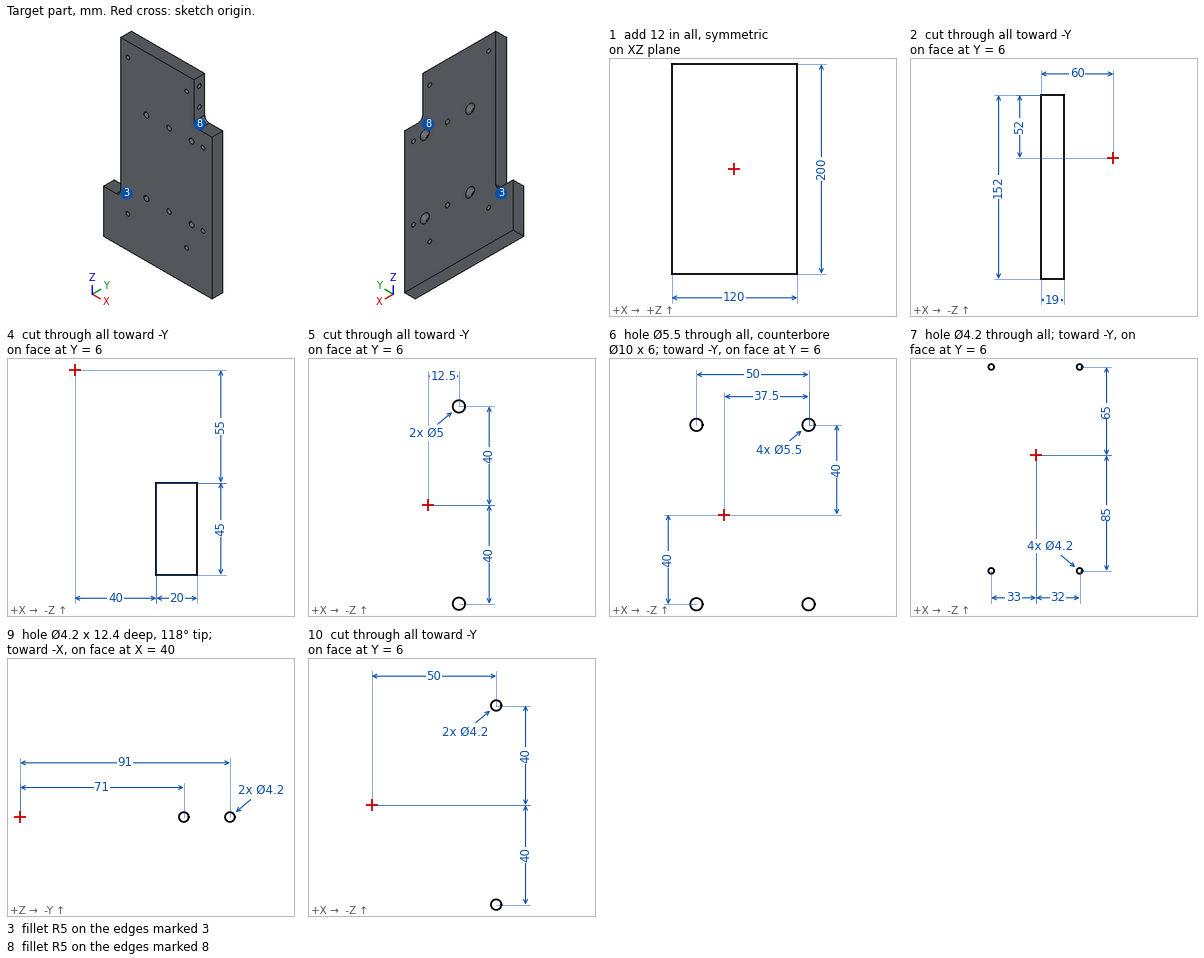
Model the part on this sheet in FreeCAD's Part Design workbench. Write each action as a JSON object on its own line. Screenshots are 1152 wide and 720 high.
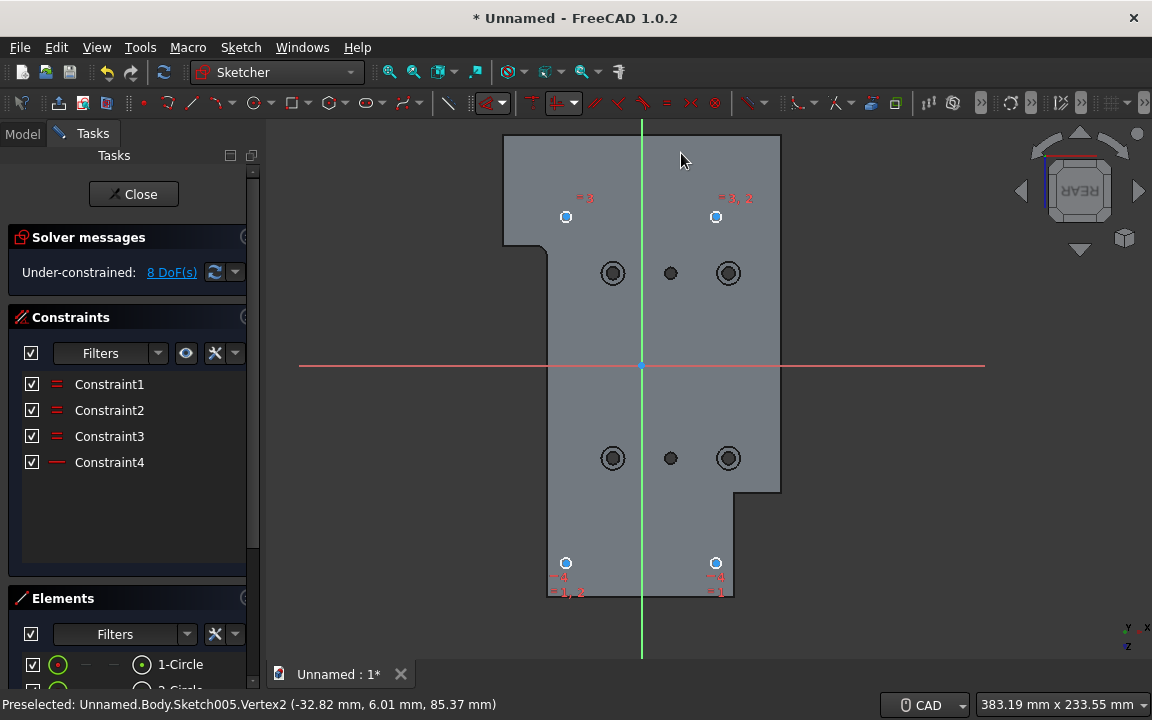
{"action": "left_click", "coordinate": [716, 563]}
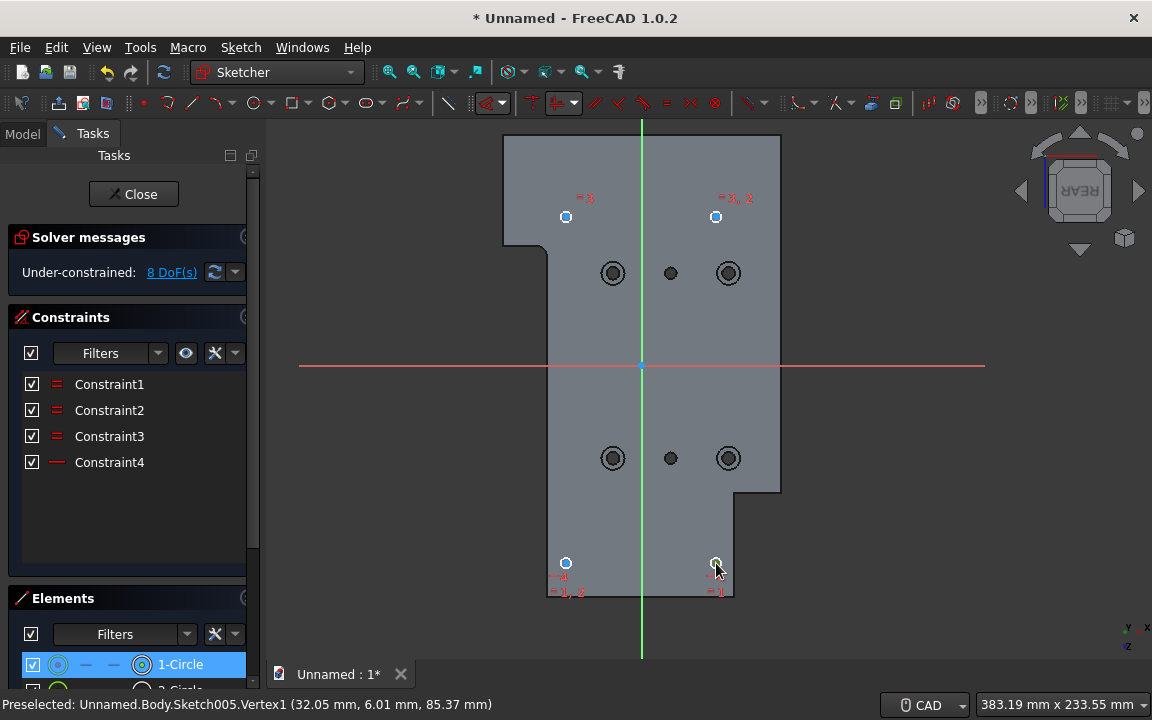
{"action": "left_click", "coordinate": [716, 217]}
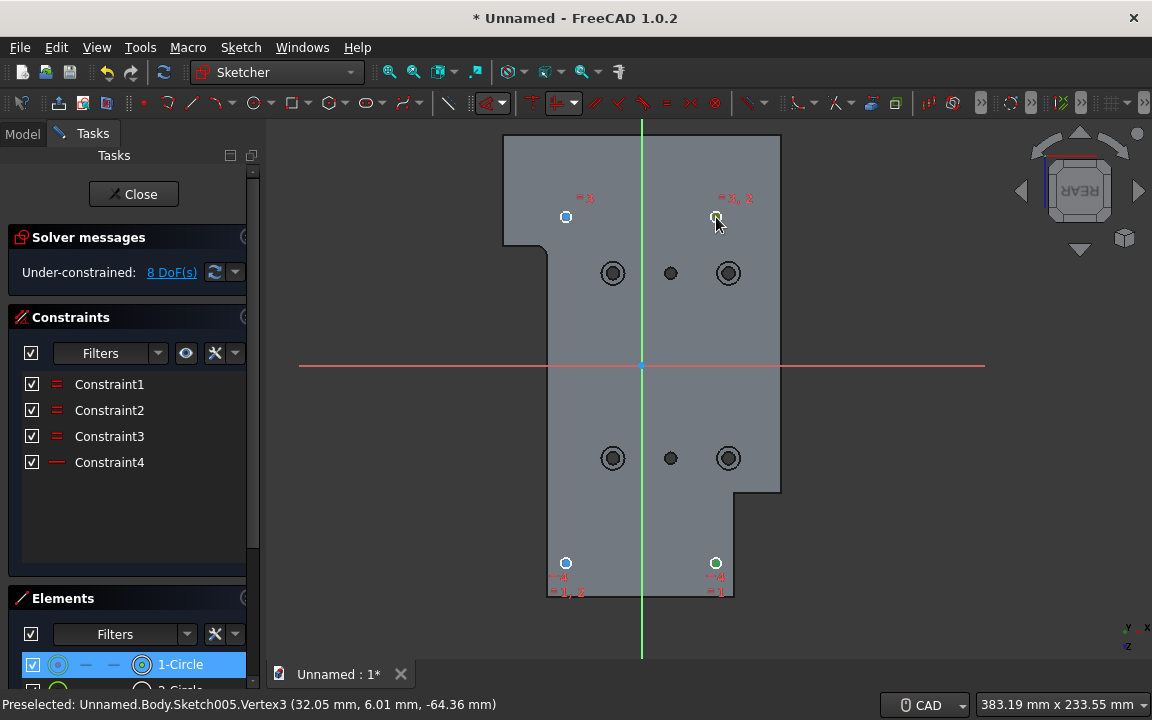
{"action": "left_click", "coordinate": [576, 104]}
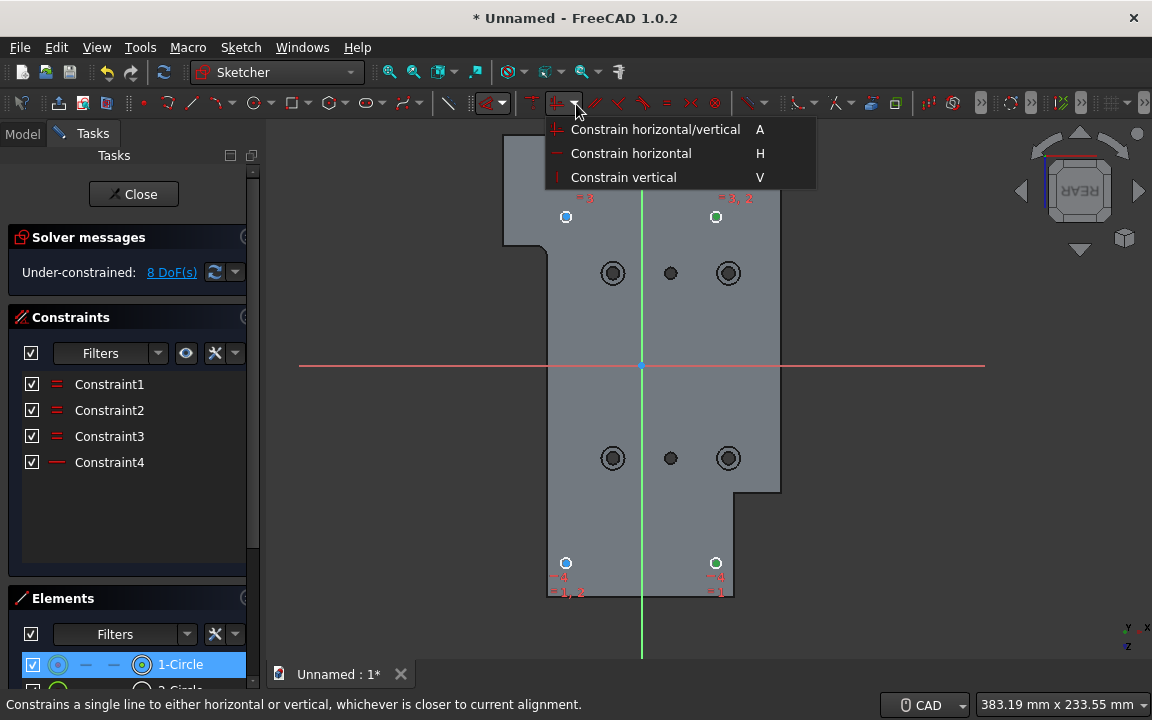
{"action": "left_click", "coordinate": [681, 177]}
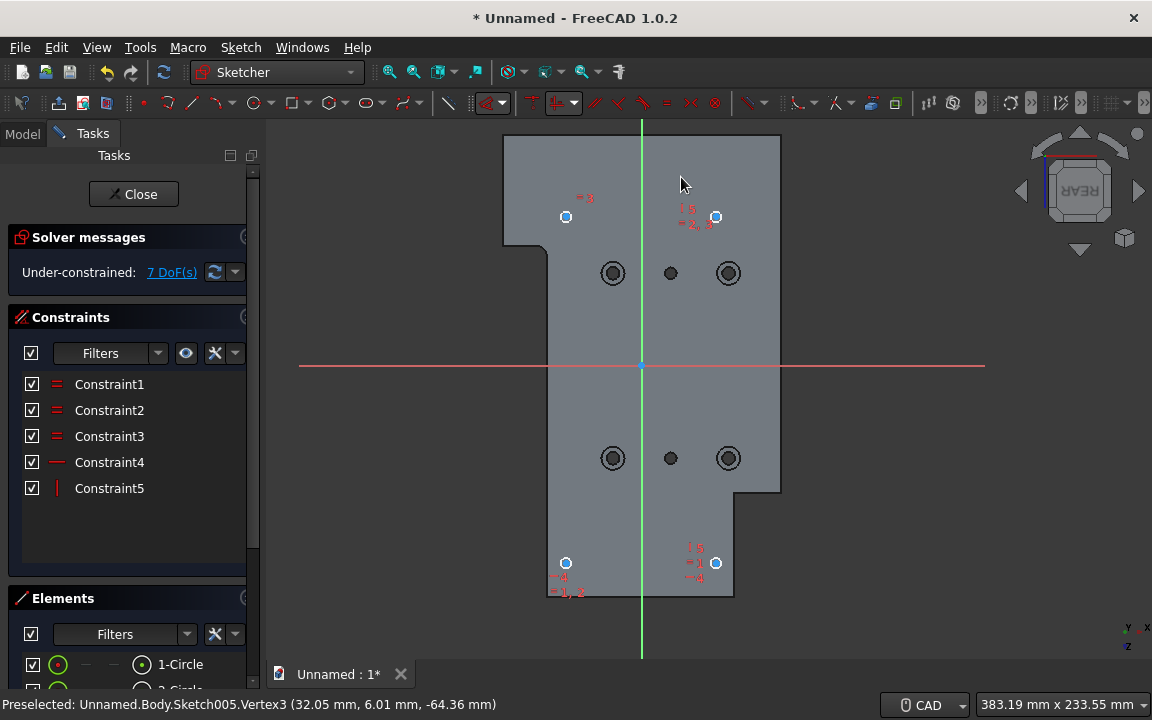
{"action": "left_click", "coordinate": [566, 563]}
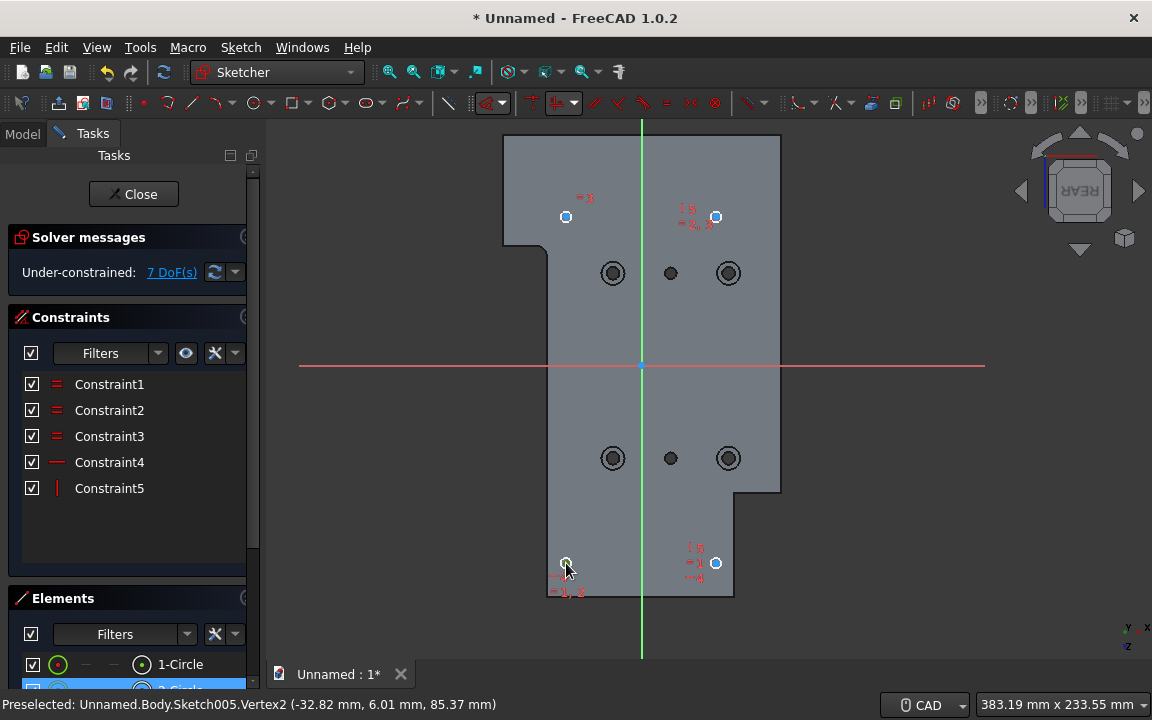
{"action": "left_click", "coordinate": [566, 217]}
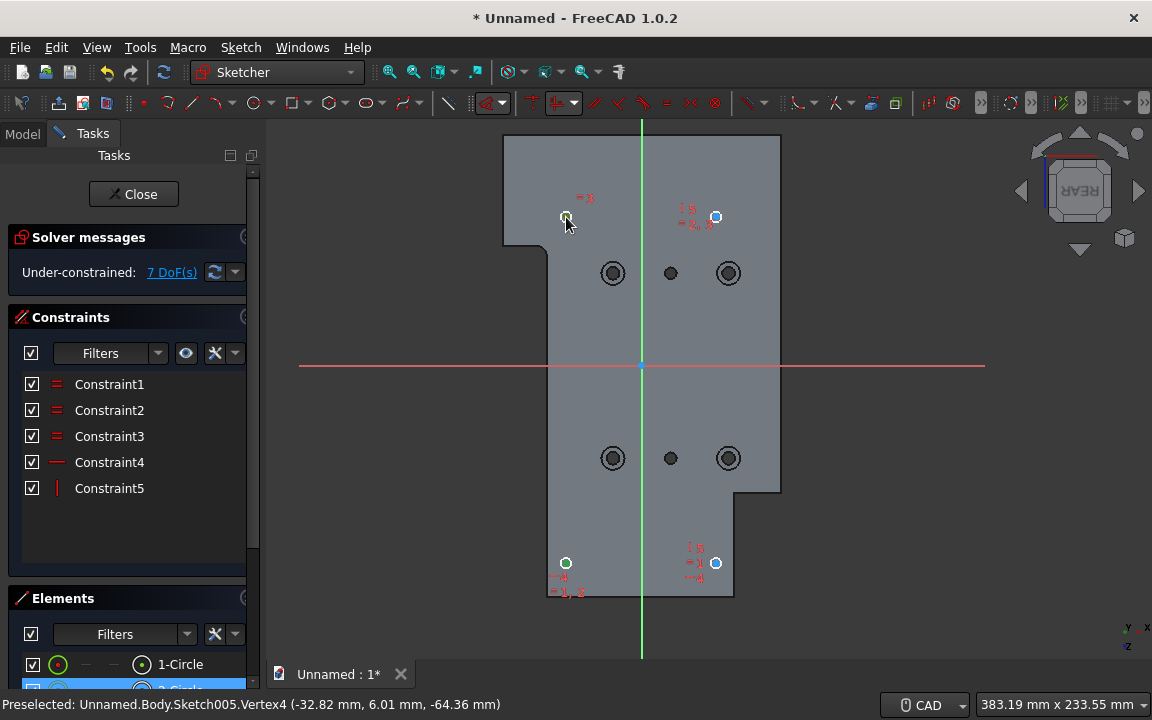
{"action": "key", "text": "v"}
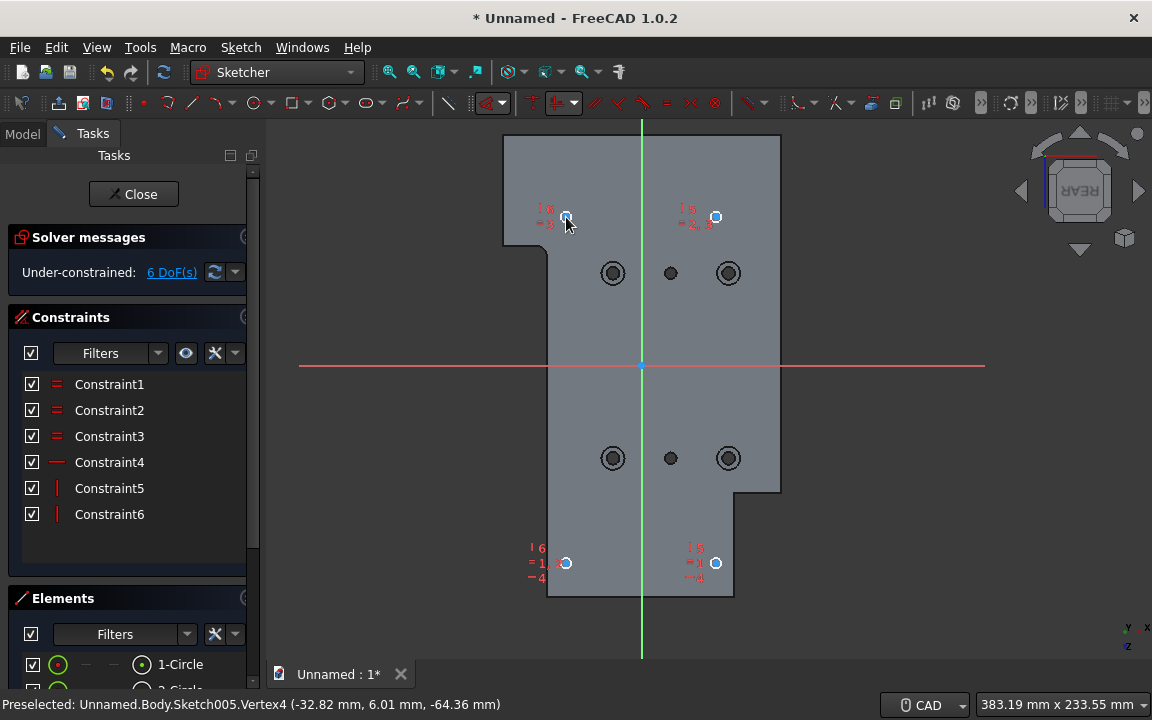
{"action": "left_click", "coordinate": [716, 217]}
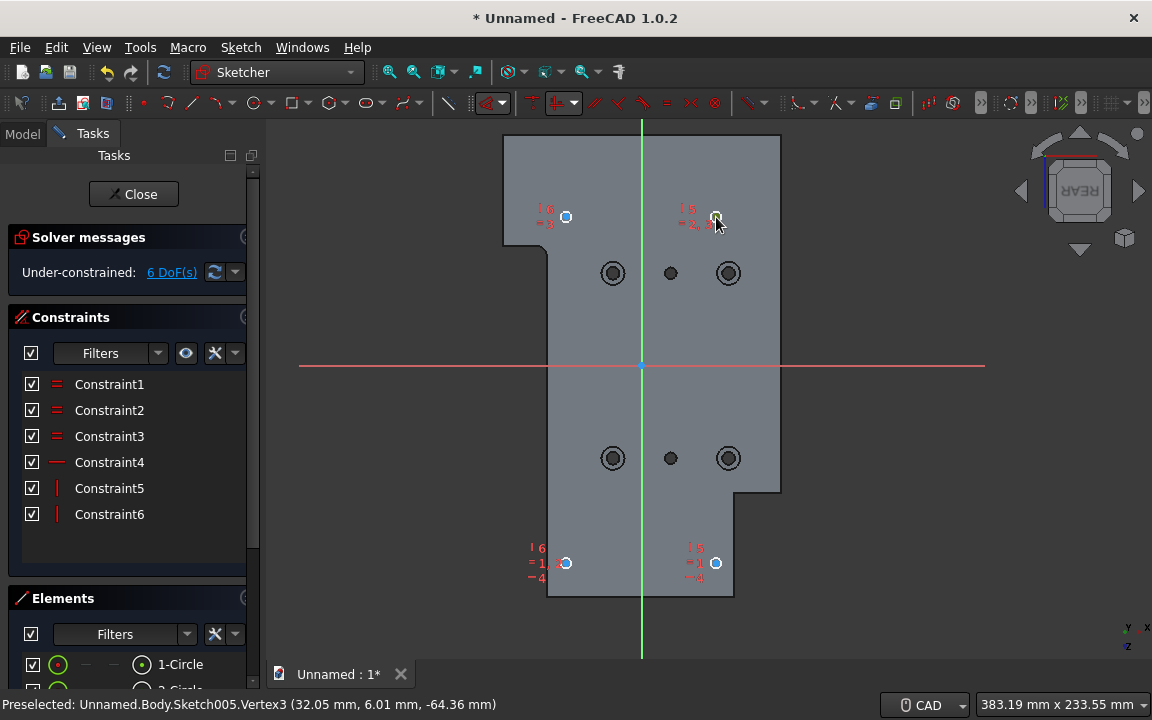
{"action": "left_click", "coordinate": [566, 217]}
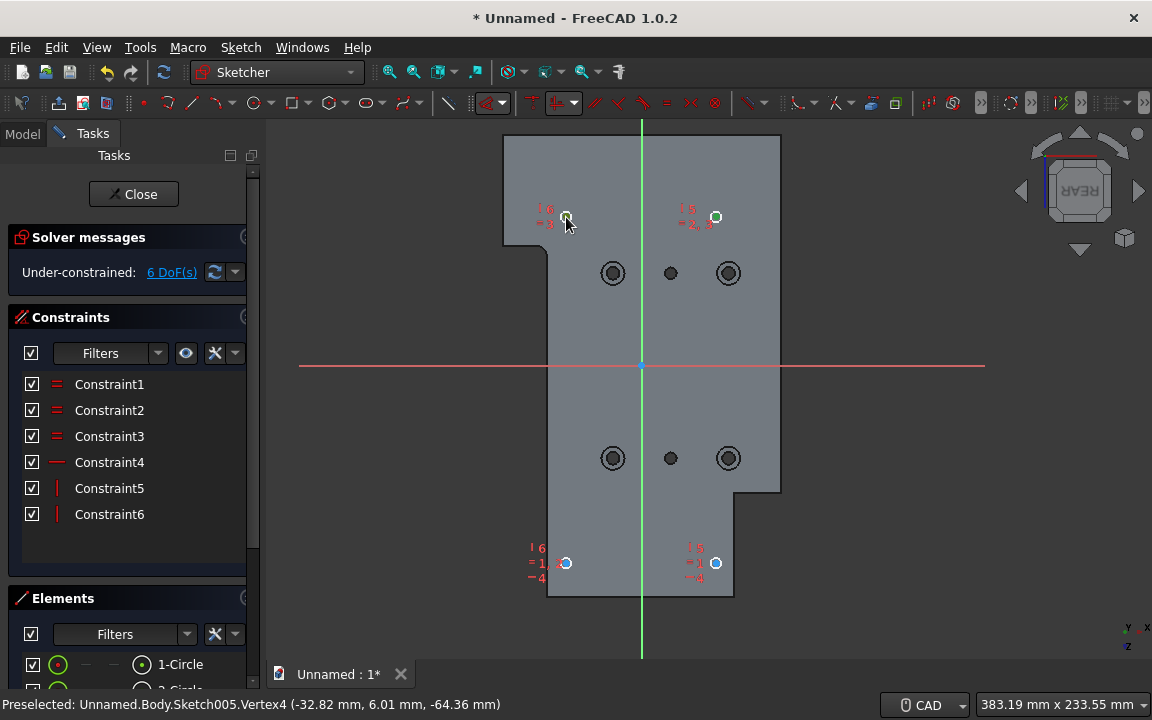
{"action": "key", "text": "h"}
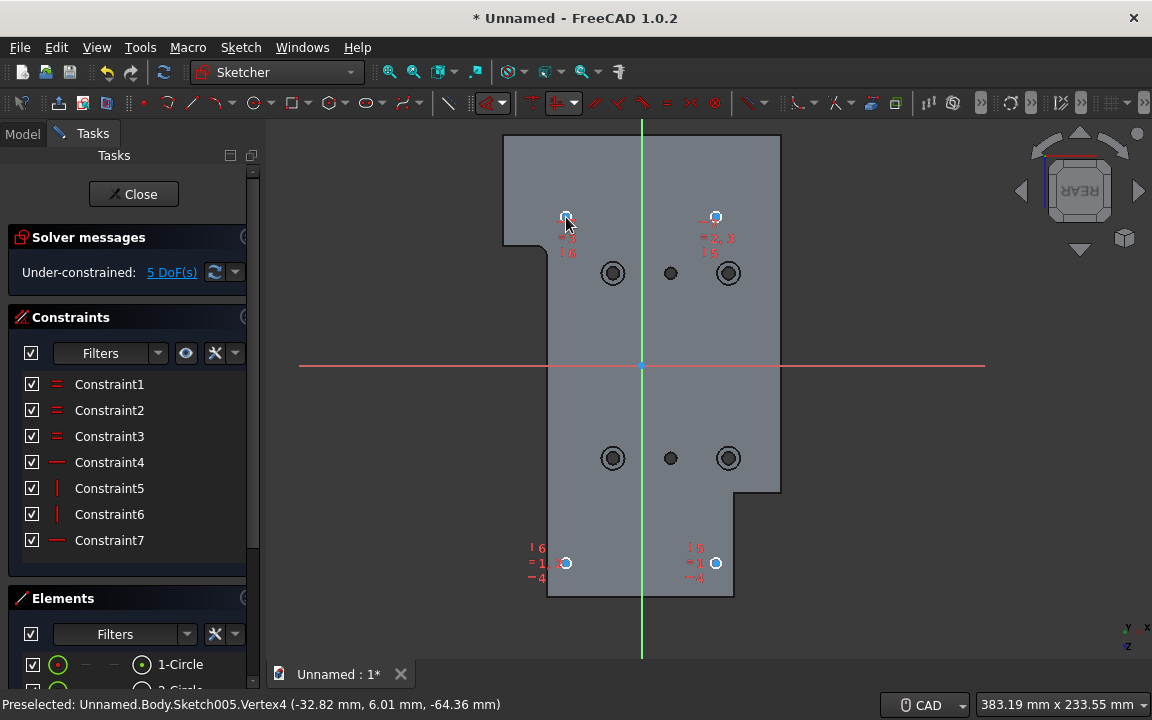
{"action": "scroll", "coordinate": [712, 560], "scroll_direction": "up", "scroll_amount": 8}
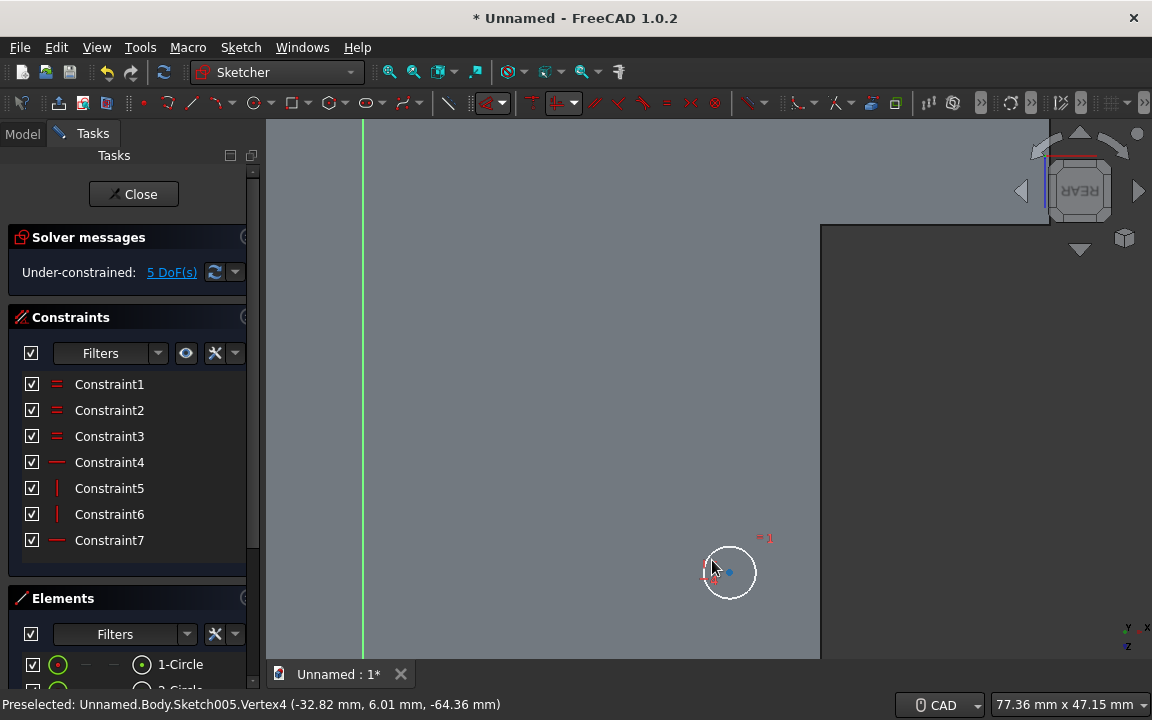
{"action": "left_click", "coordinate": [711, 554]}